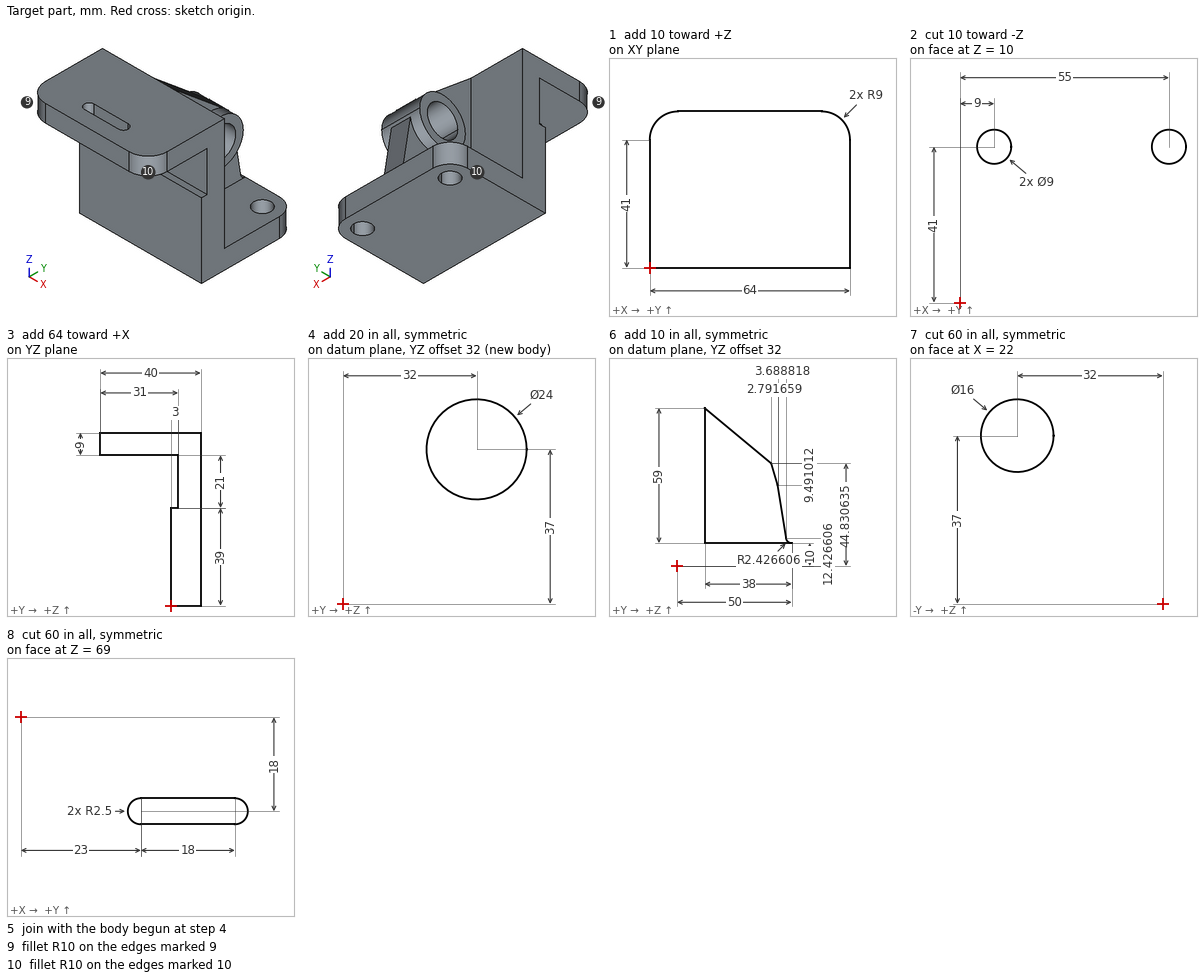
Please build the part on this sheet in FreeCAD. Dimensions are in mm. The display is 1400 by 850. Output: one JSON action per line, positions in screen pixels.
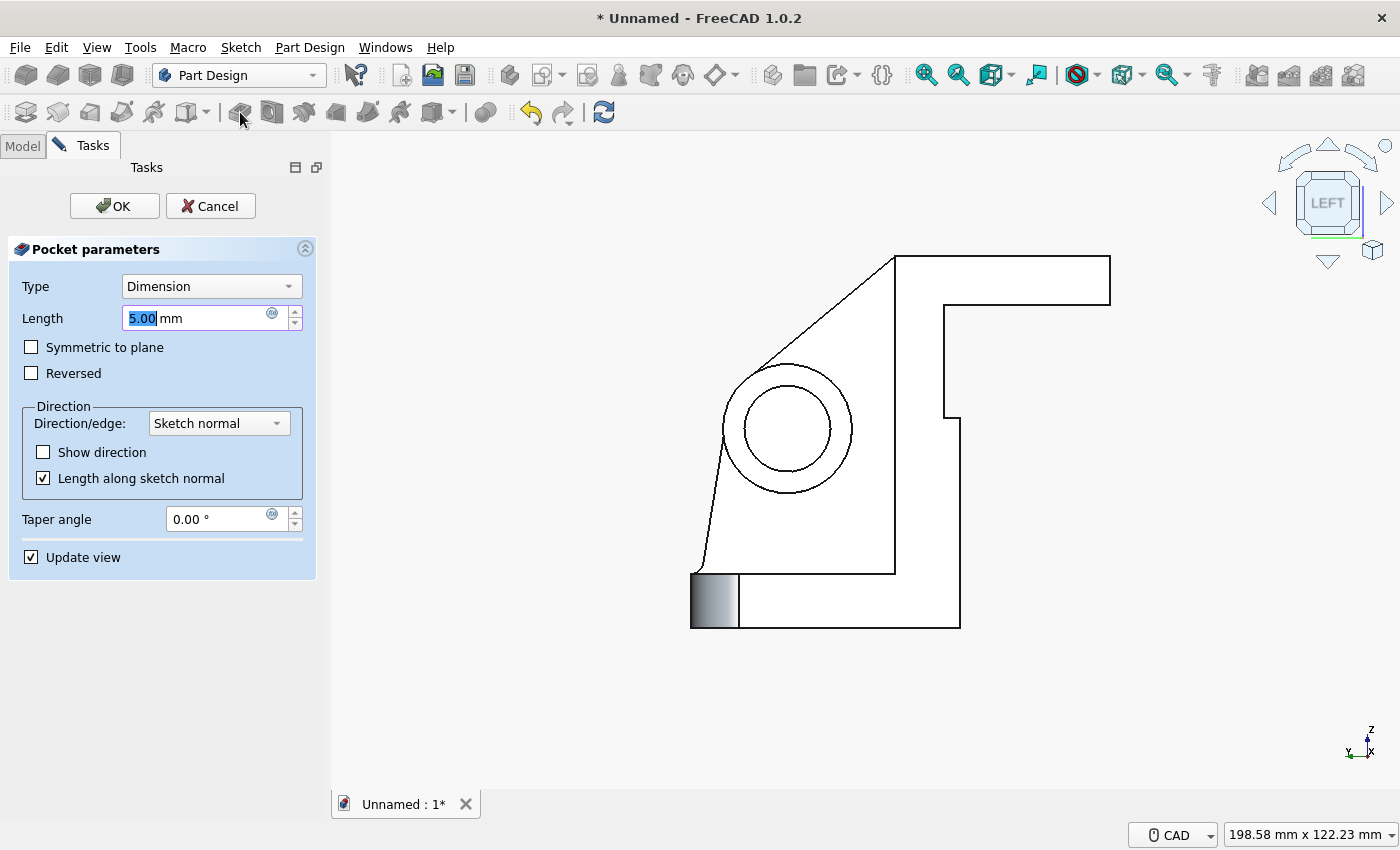
{"action": "type", "text": "60"}
{"action": "key", "text": "Tab"}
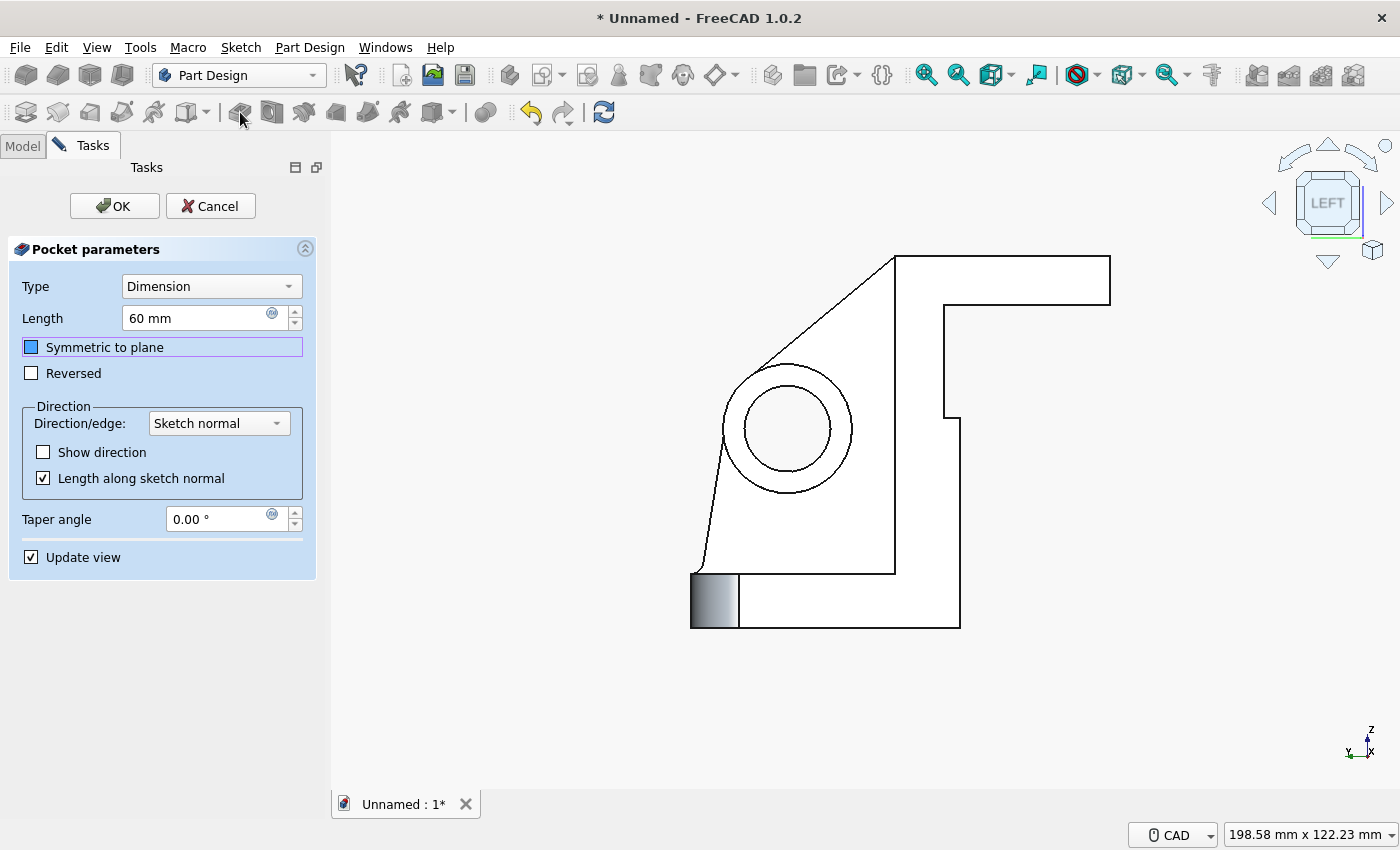
{"action": "left_click", "coordinate": [30, 347]}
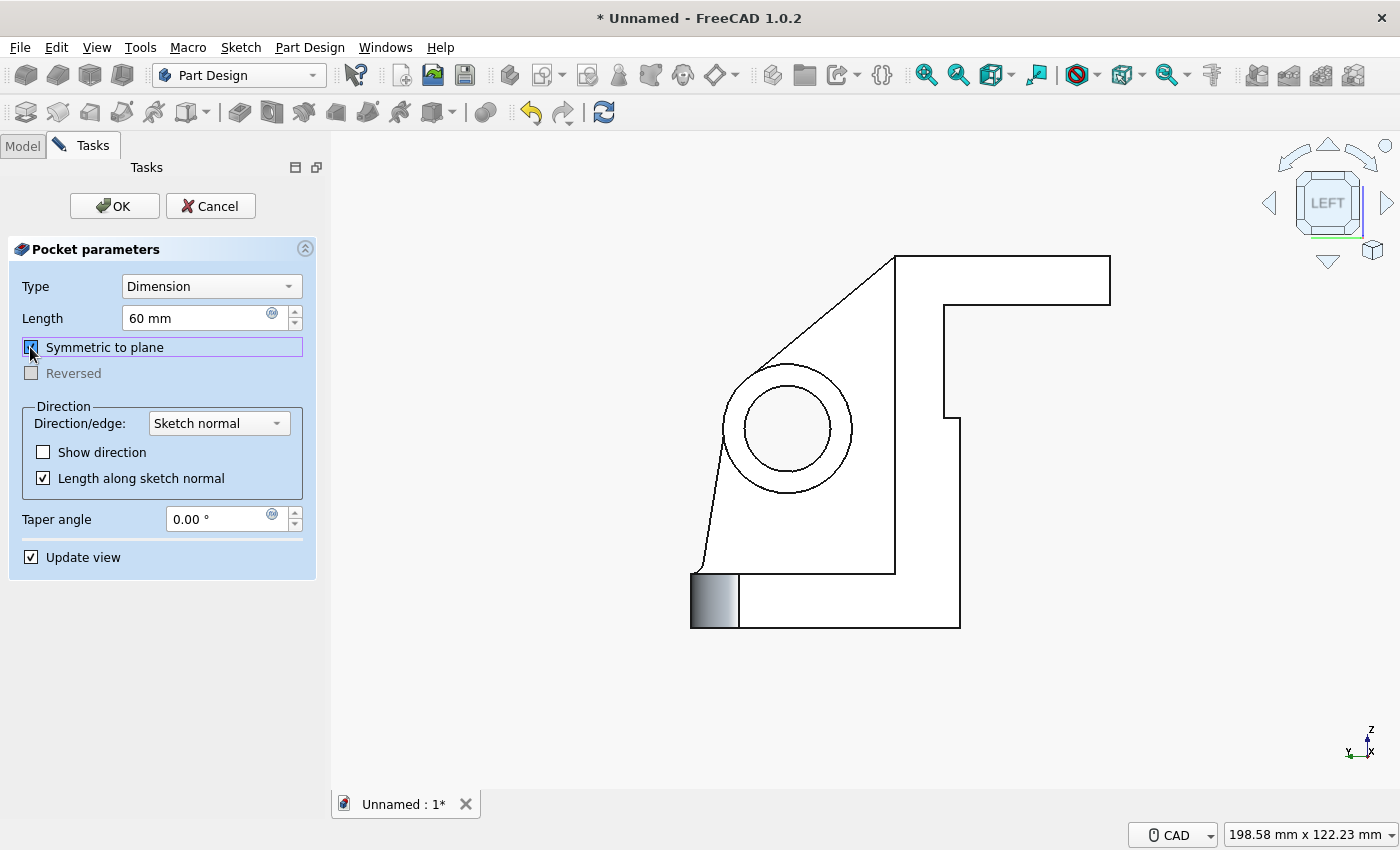
{"action": "left_click", "coordinate": [115, 206]}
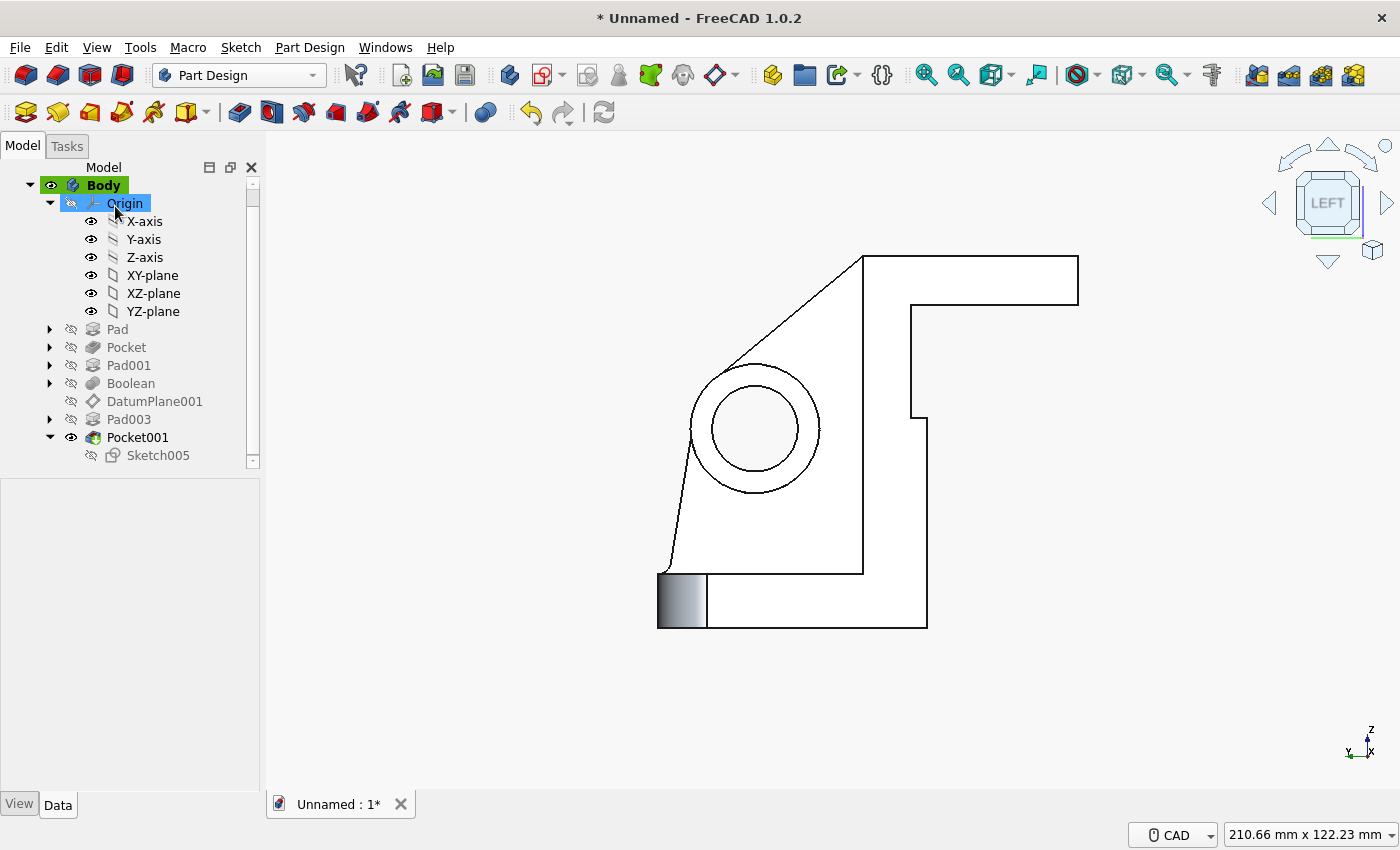
{"action": "key", "text": "0"}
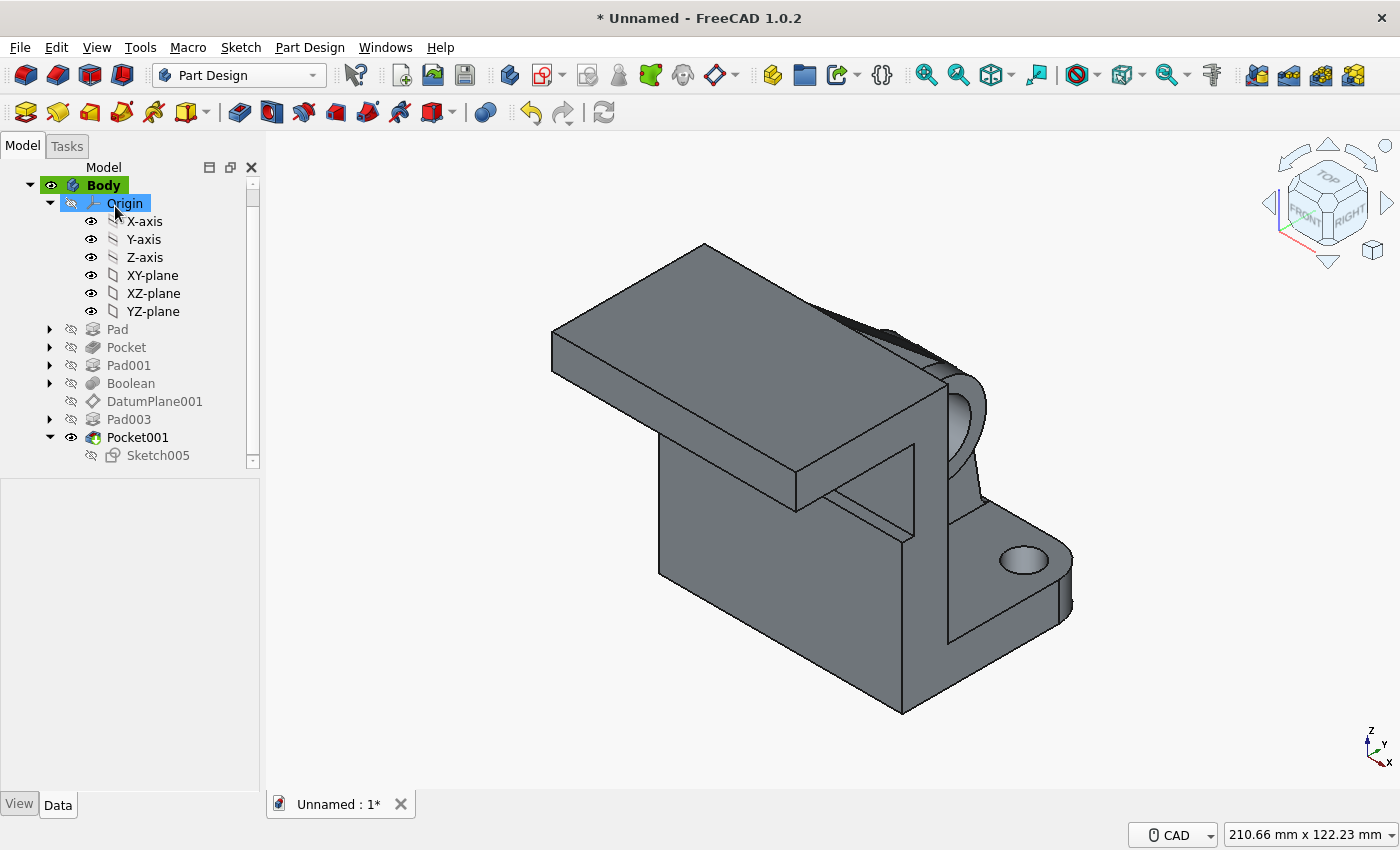
{"action": "left_click", "coordinate": [785, 377]}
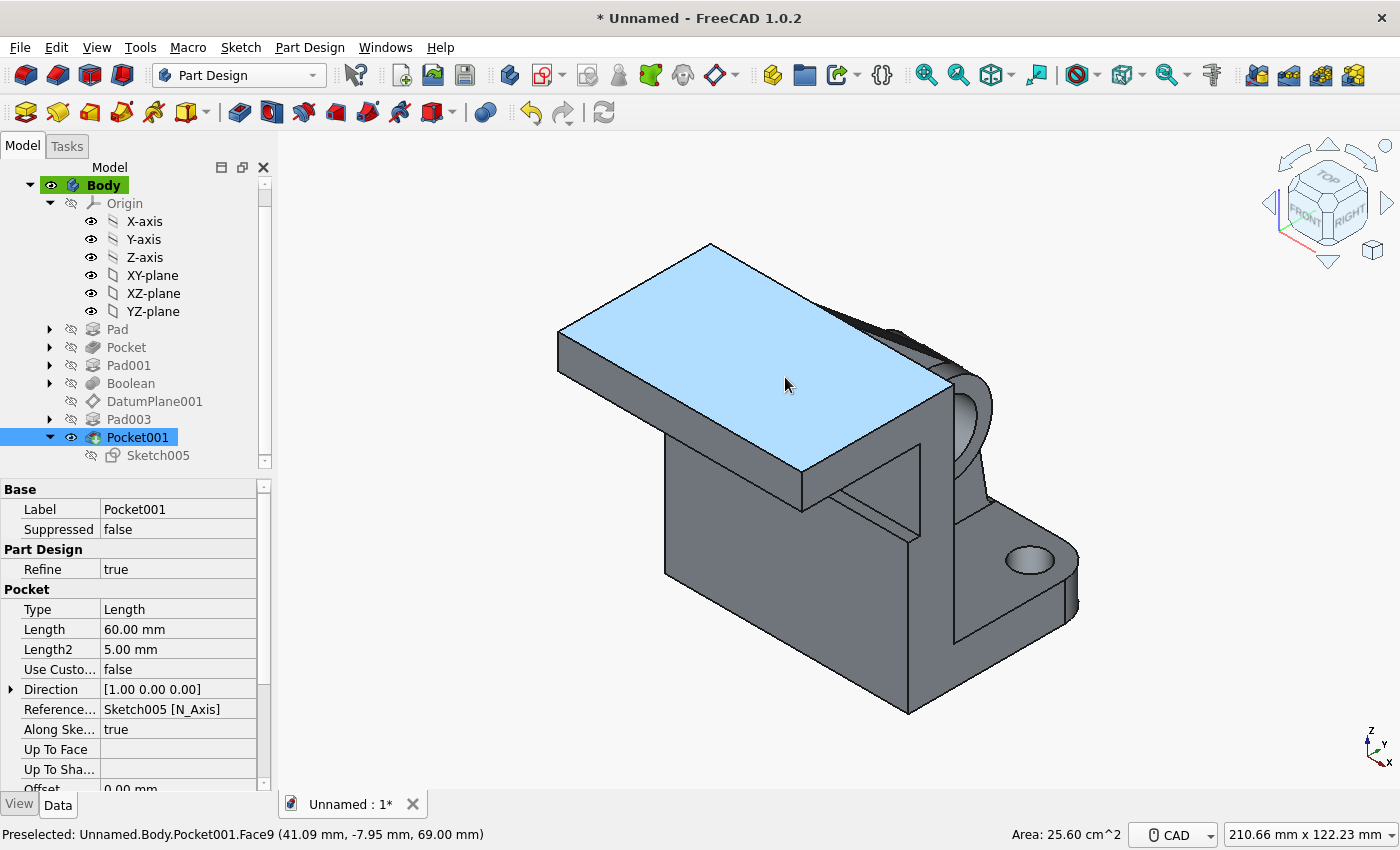
{"action": "left_click", "coordinate": [542, 76]}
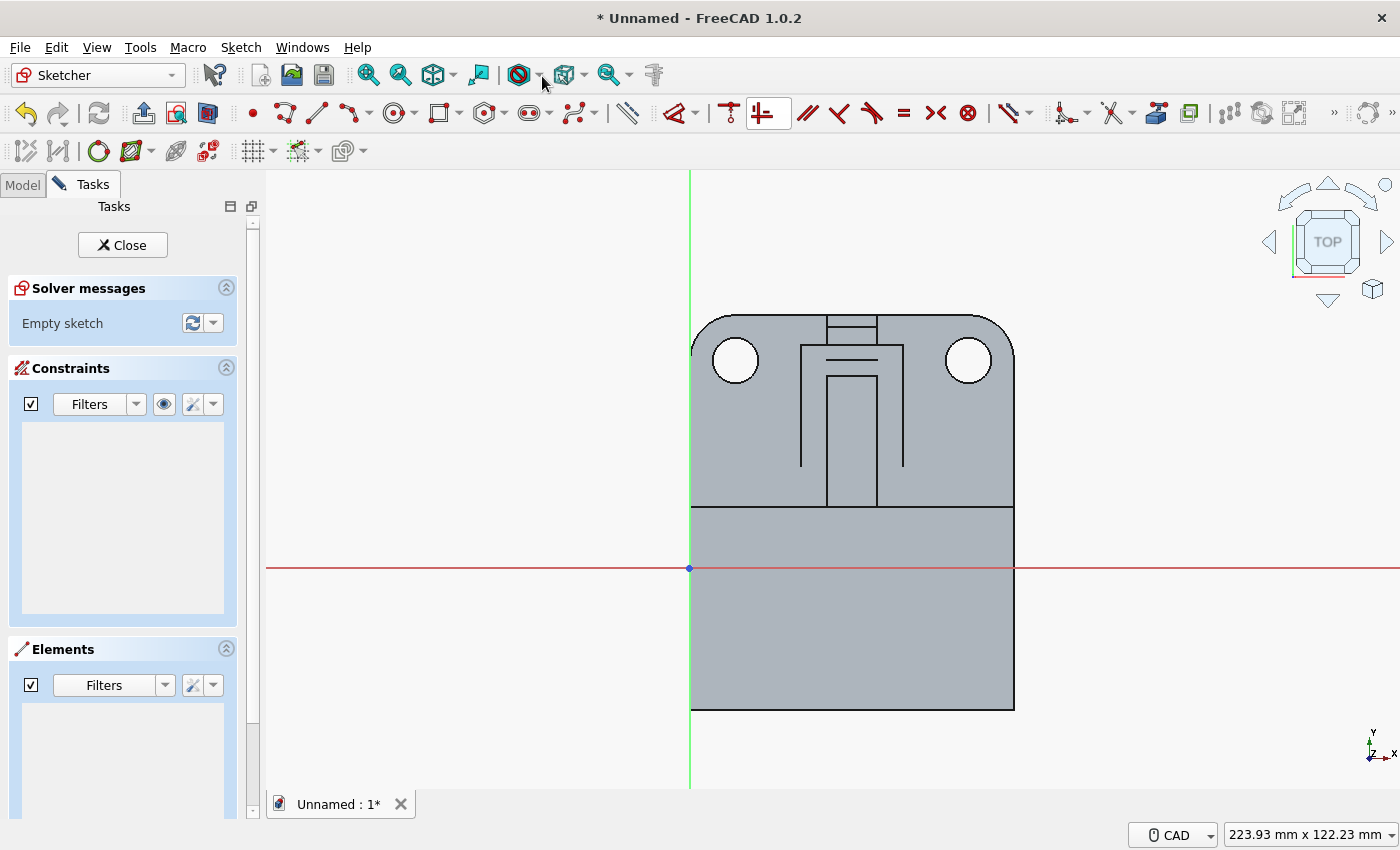
{"action": "scroll", "coordinate": [815, 681], "scroll_direction": "up", "scroll_amount": 6}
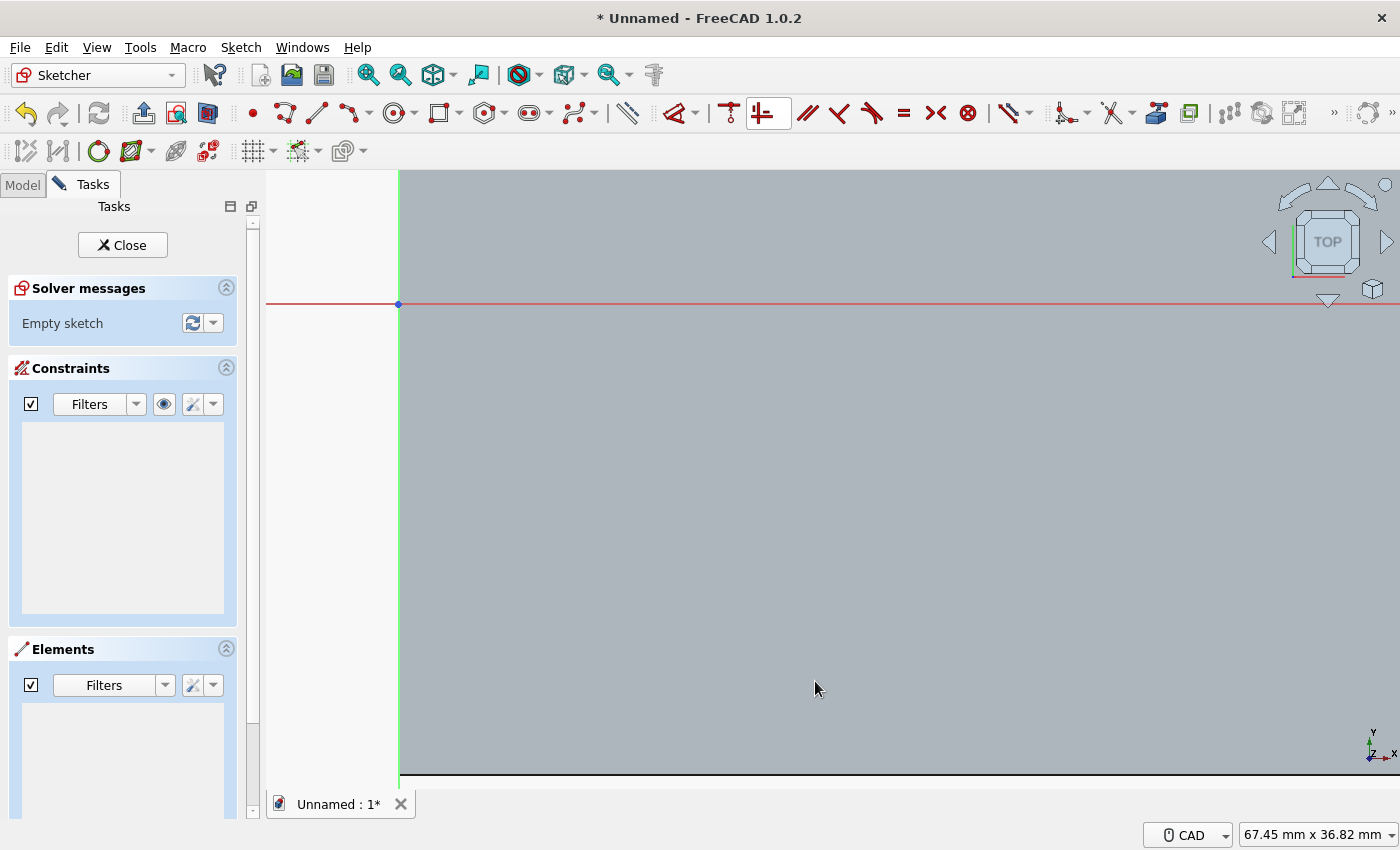
{"action": "left_click", "coordinate": [530, 114]}